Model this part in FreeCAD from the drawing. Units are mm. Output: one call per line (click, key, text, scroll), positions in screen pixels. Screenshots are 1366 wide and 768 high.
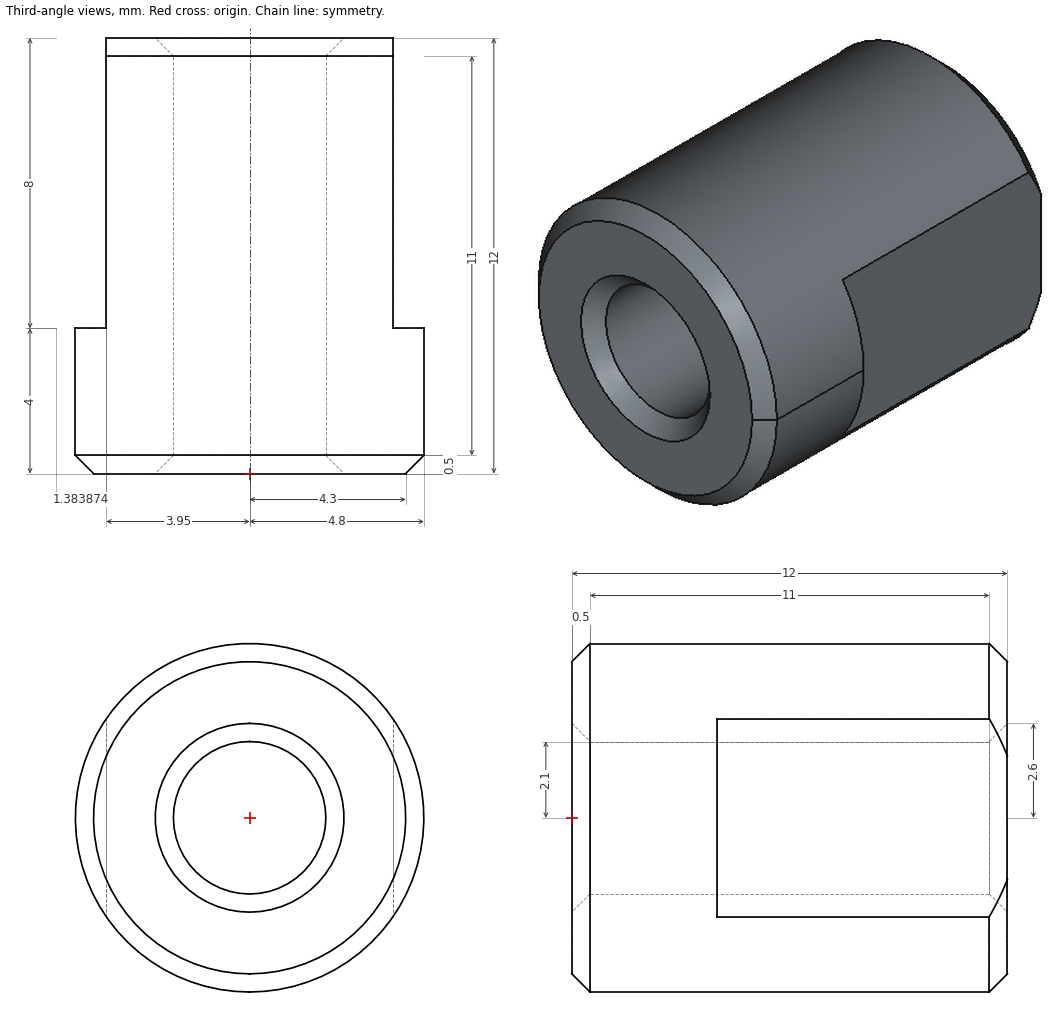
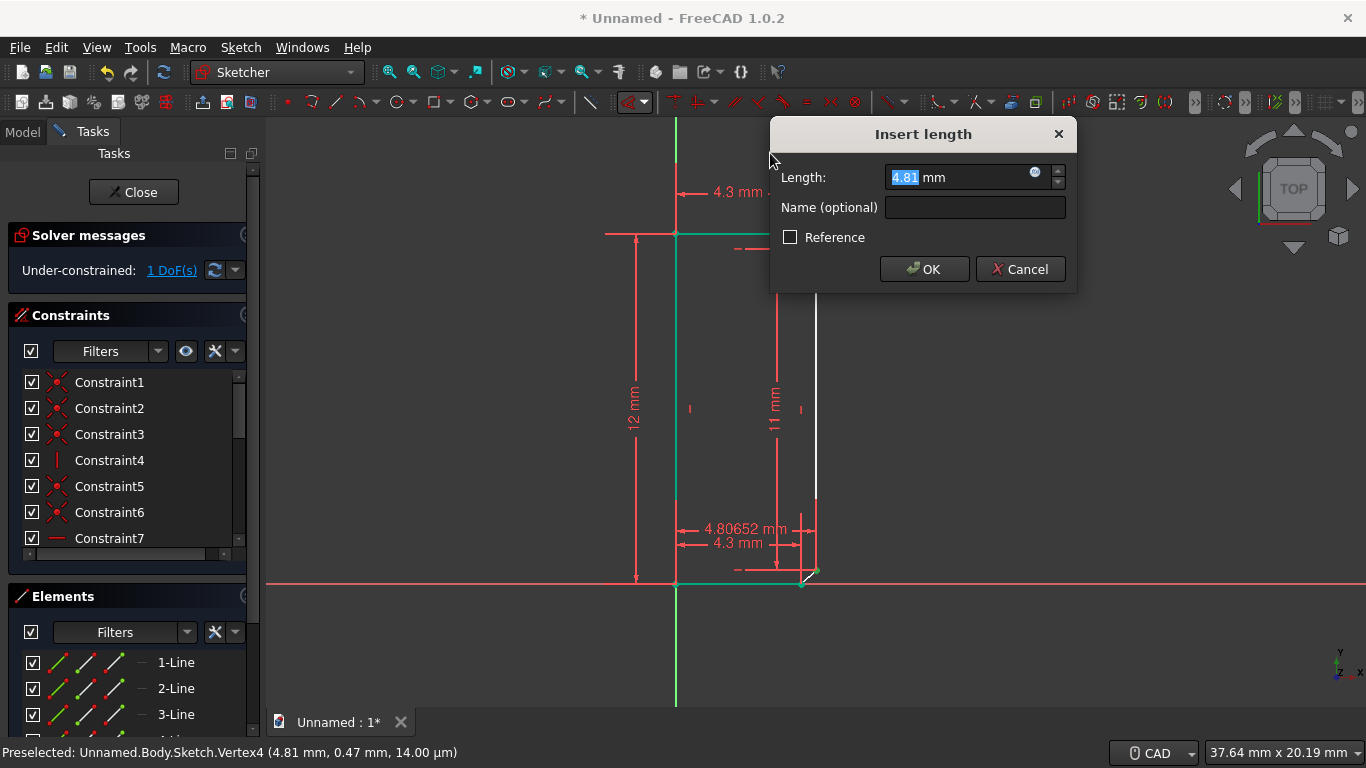
text(4.8)
key(Return)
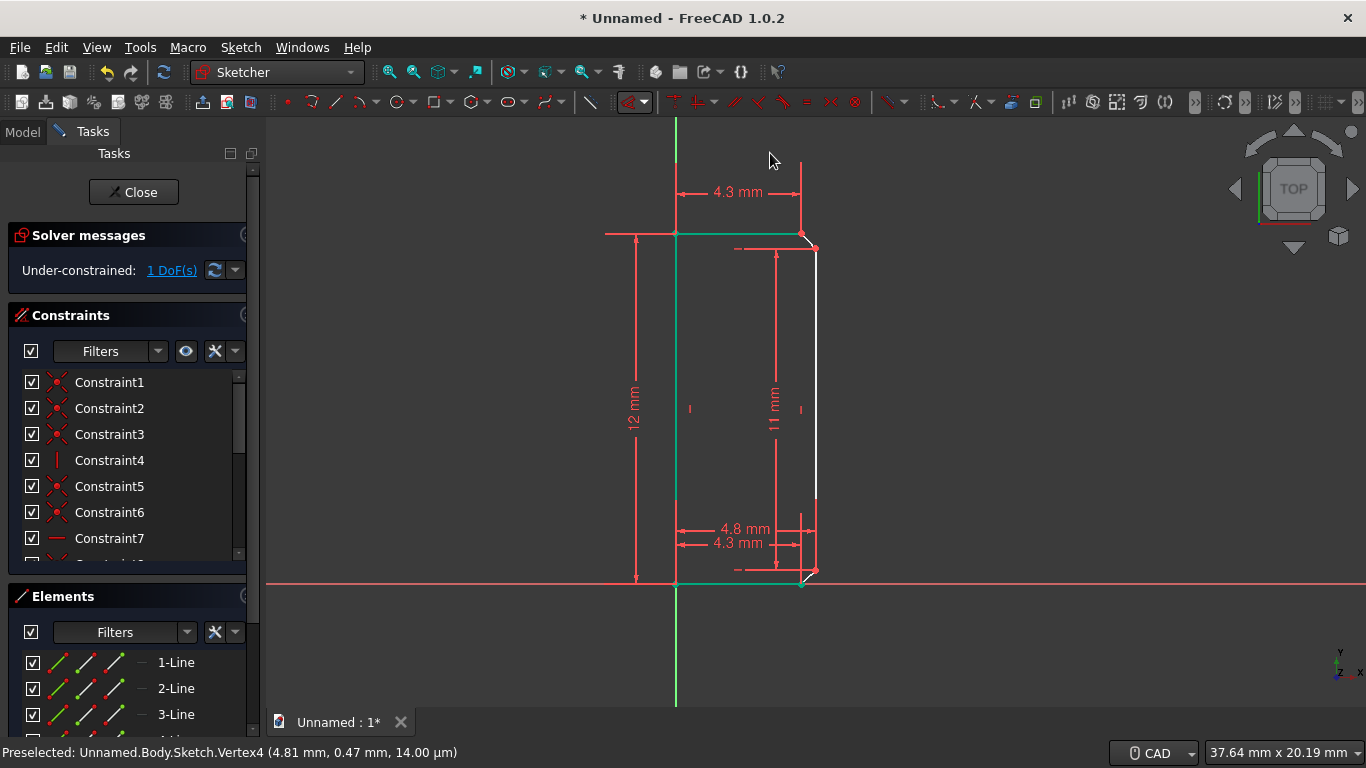
scroll(816, 570, up, 5)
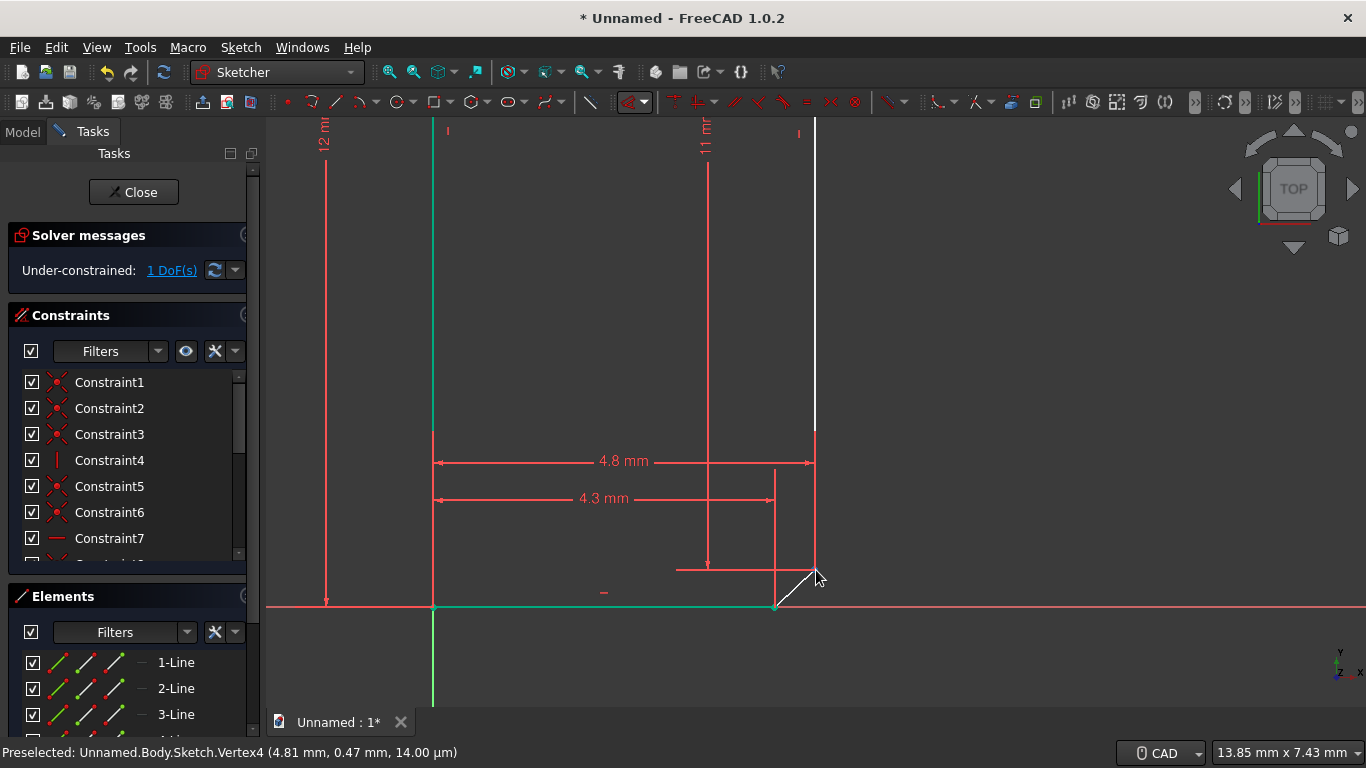
click(815, 570)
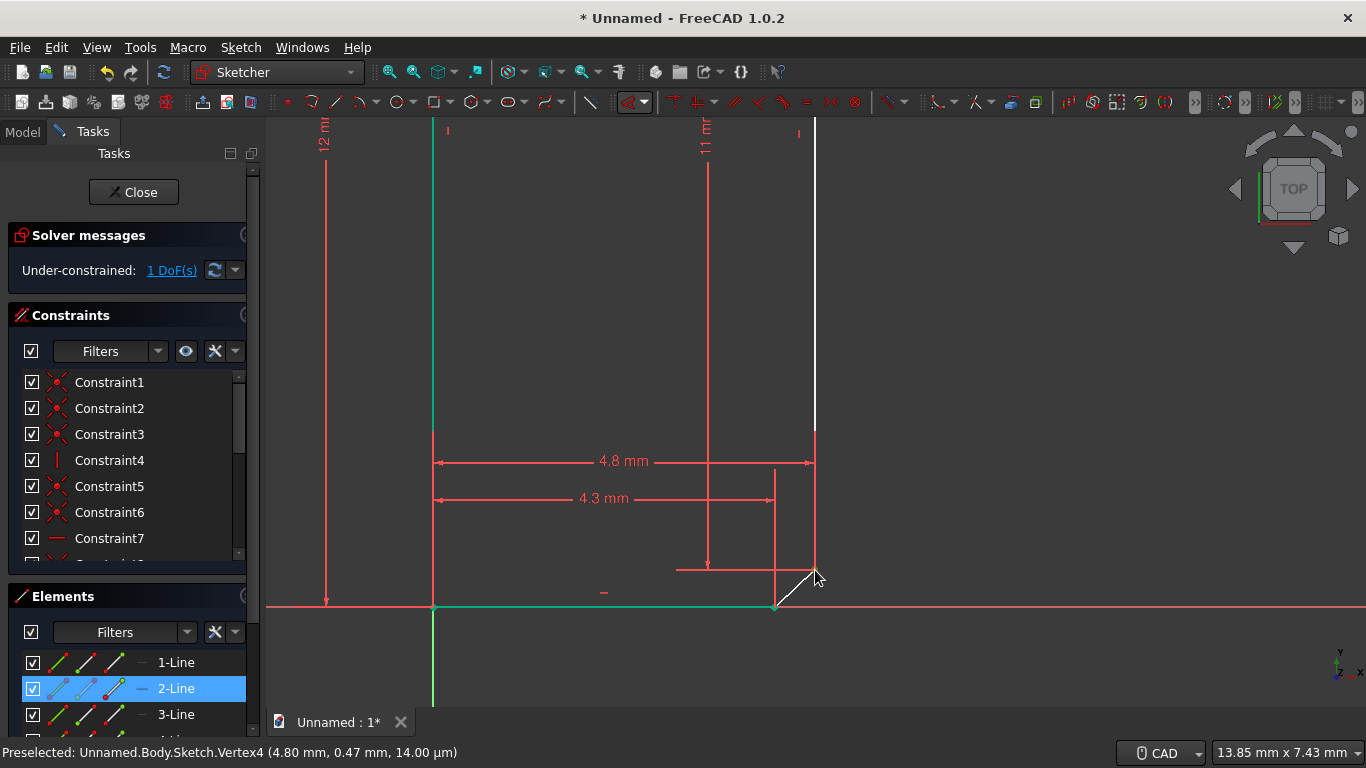
click(646, 102)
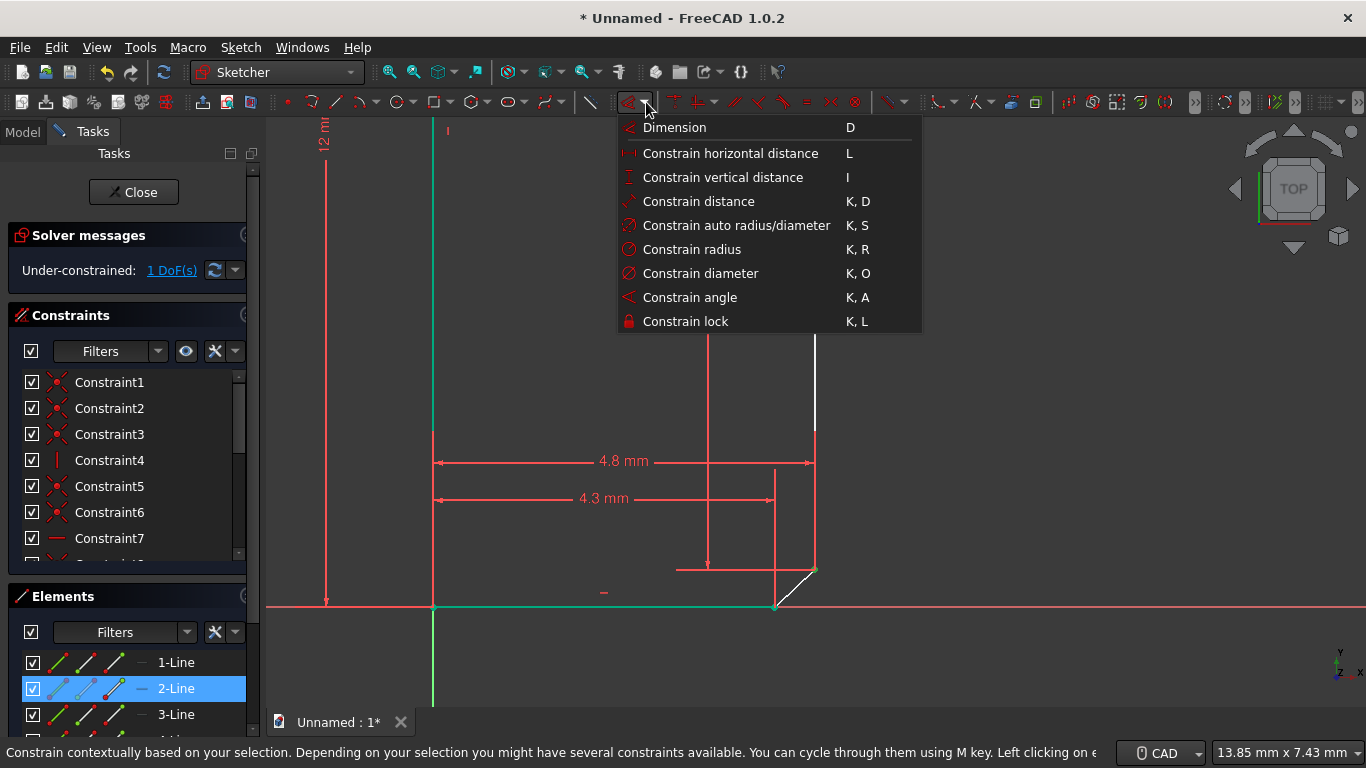
click(770, 177)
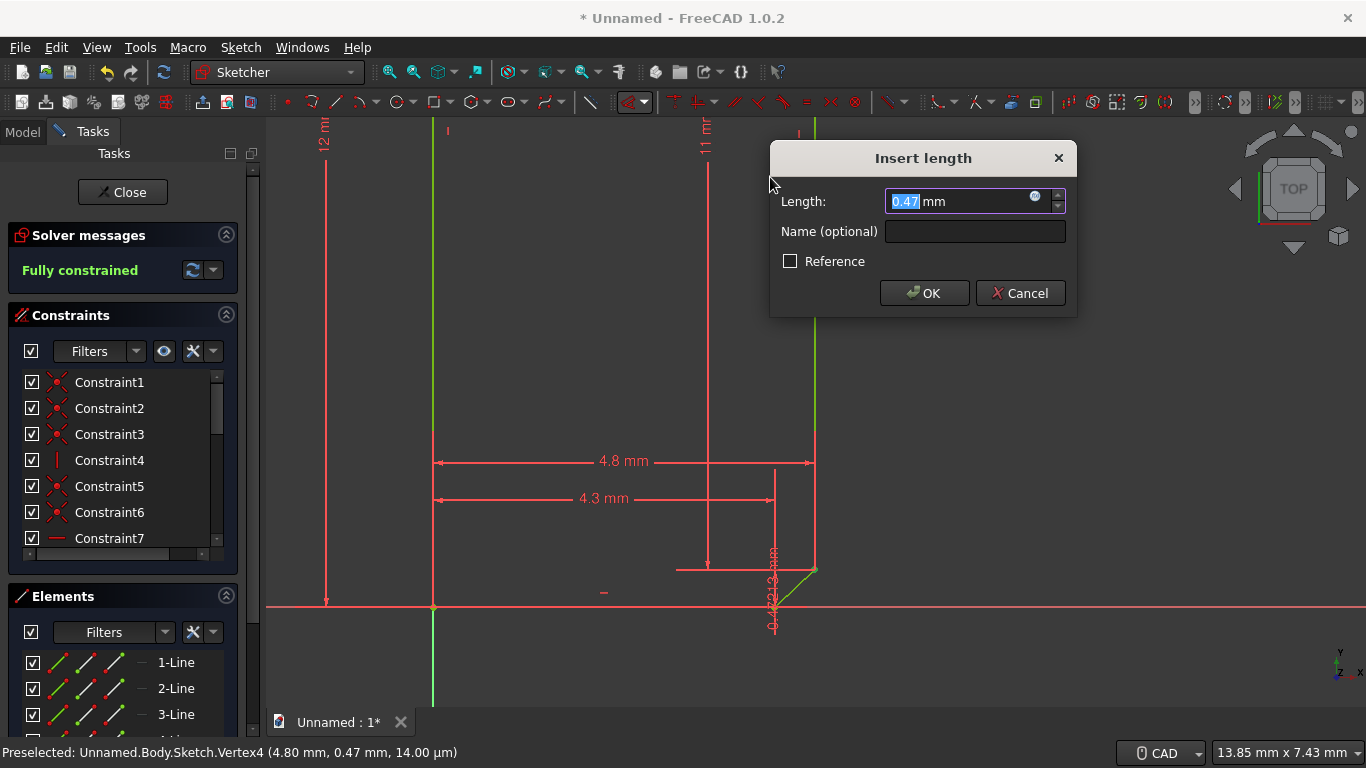
text(0.5)
key(Return)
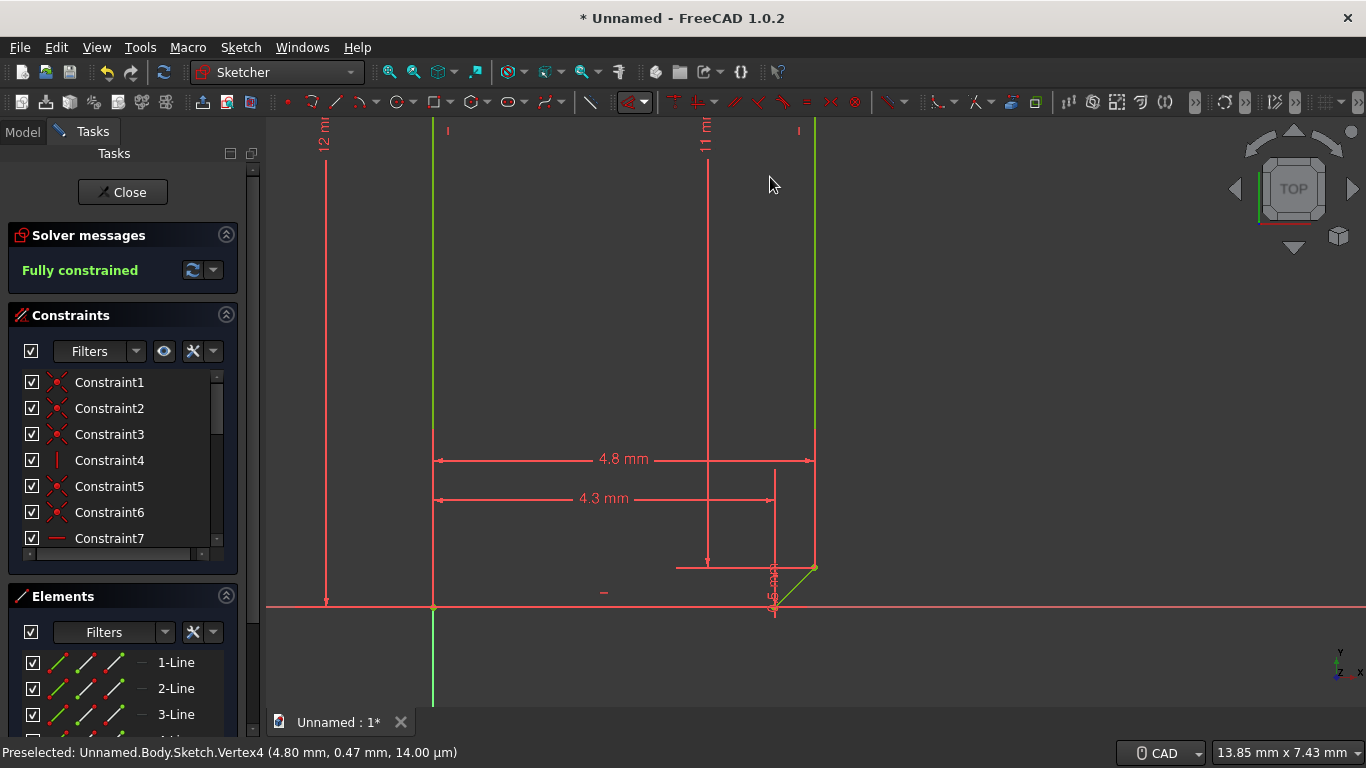
click(123, 192)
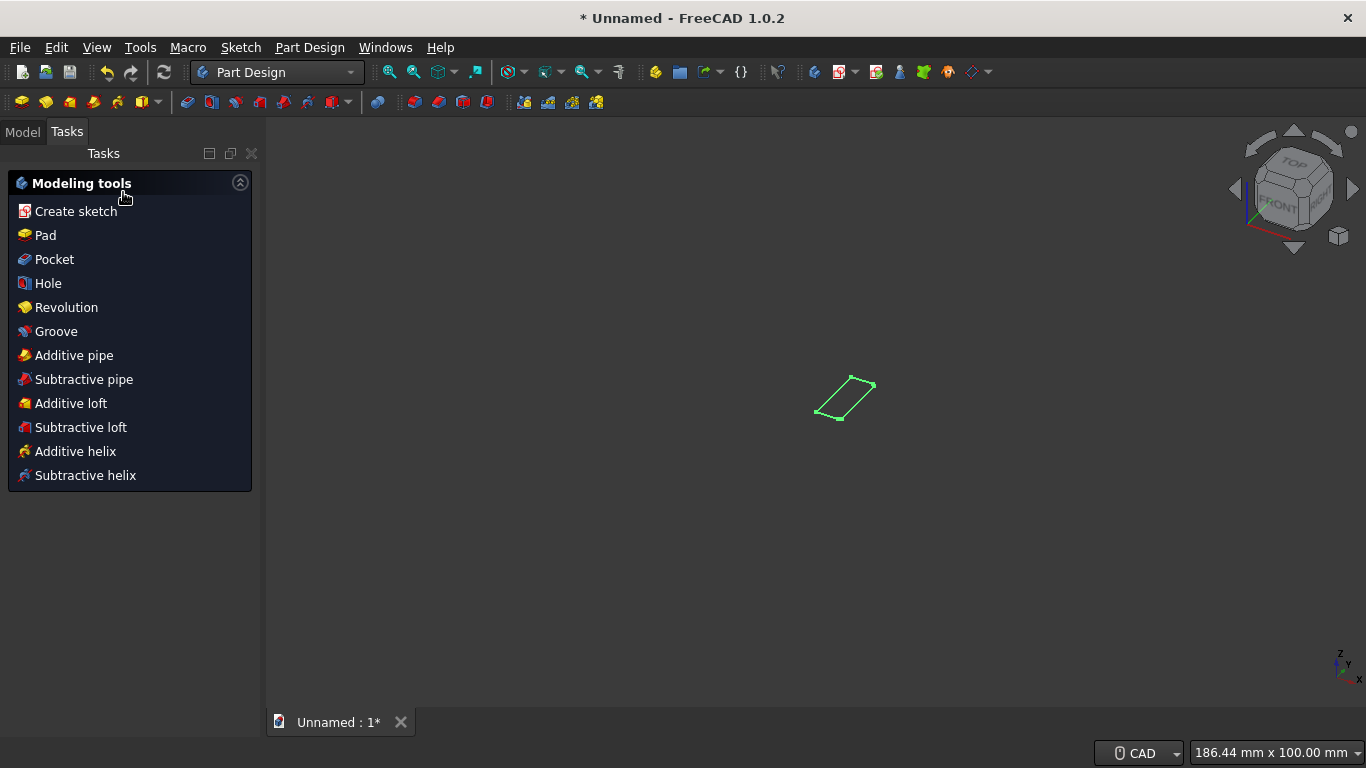
click(46, 102)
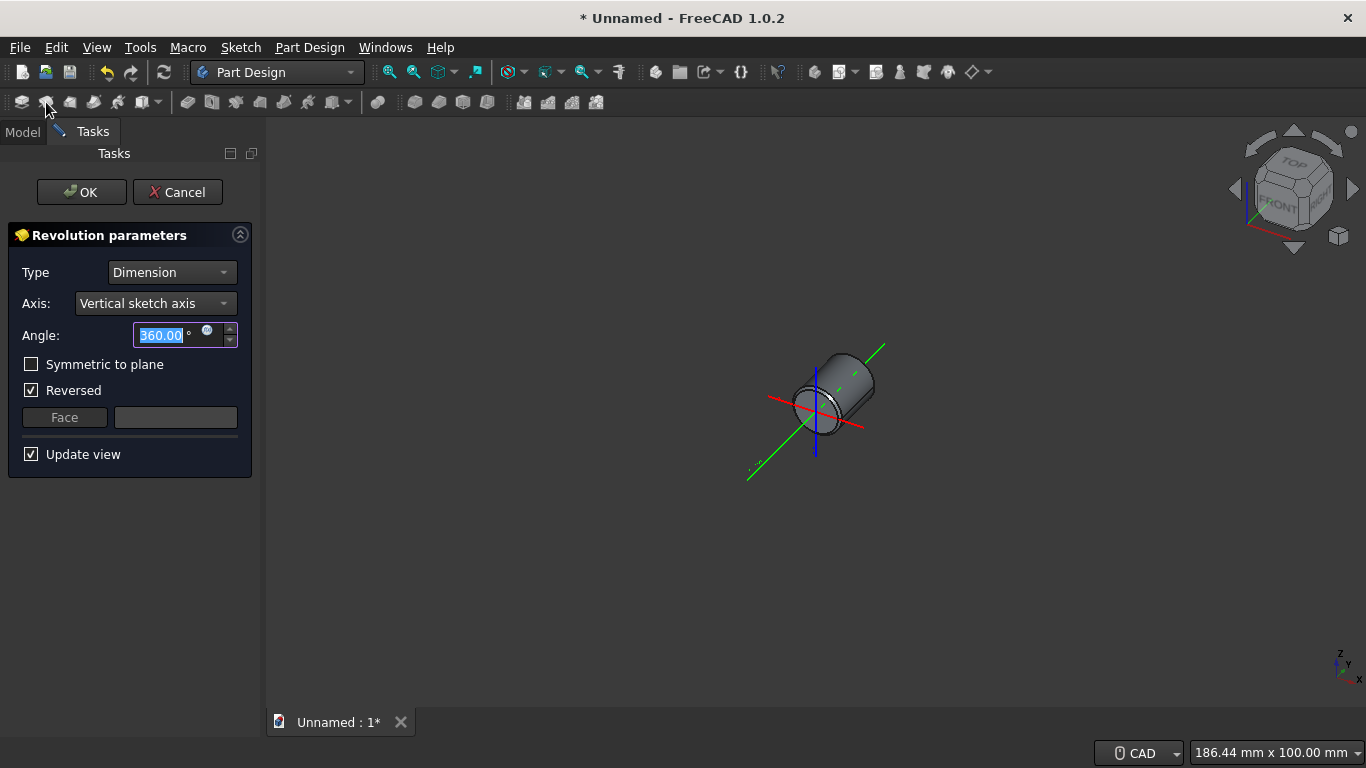
click(82, 192)